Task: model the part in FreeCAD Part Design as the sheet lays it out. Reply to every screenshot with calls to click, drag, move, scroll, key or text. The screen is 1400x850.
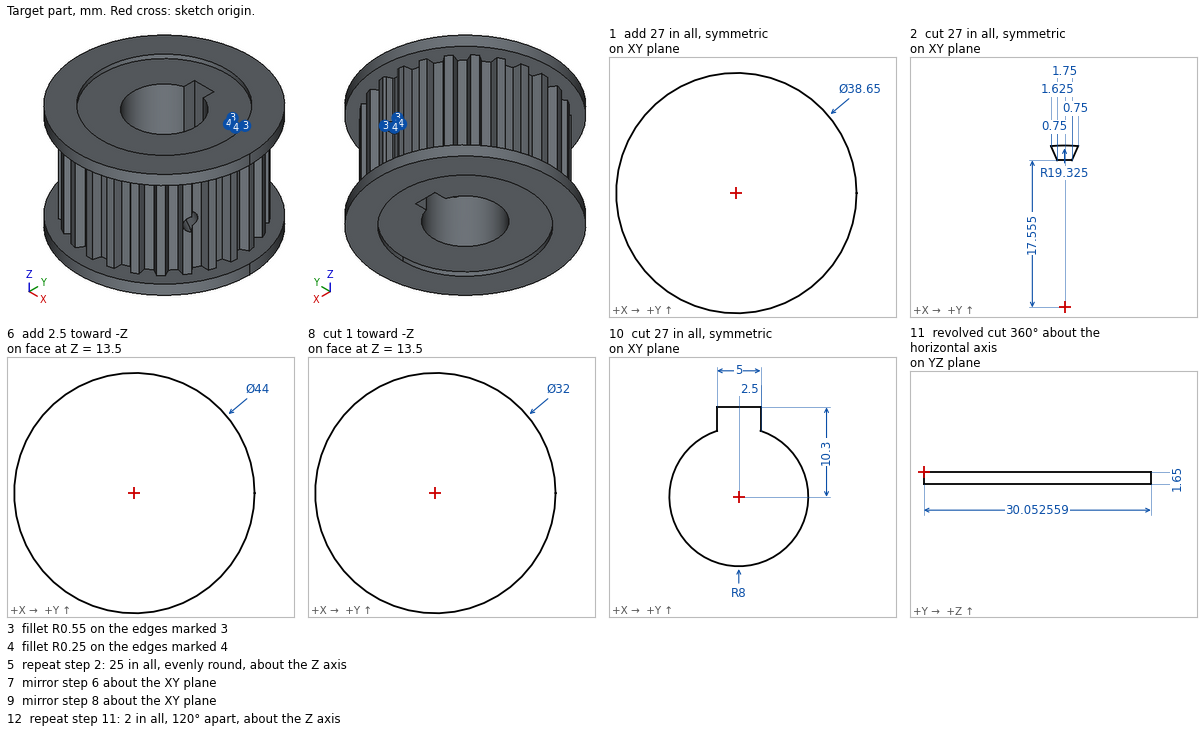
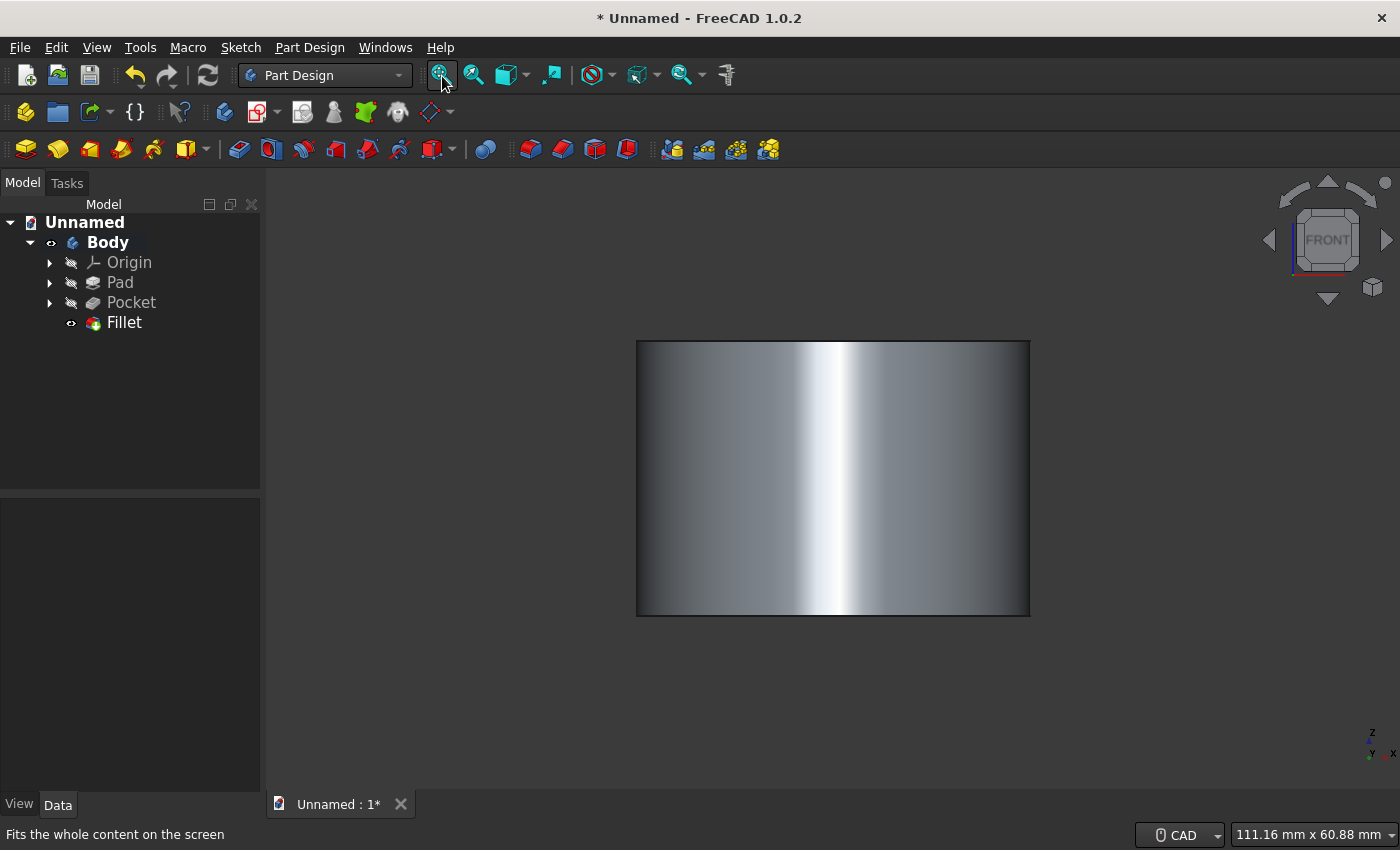
click(442, 76)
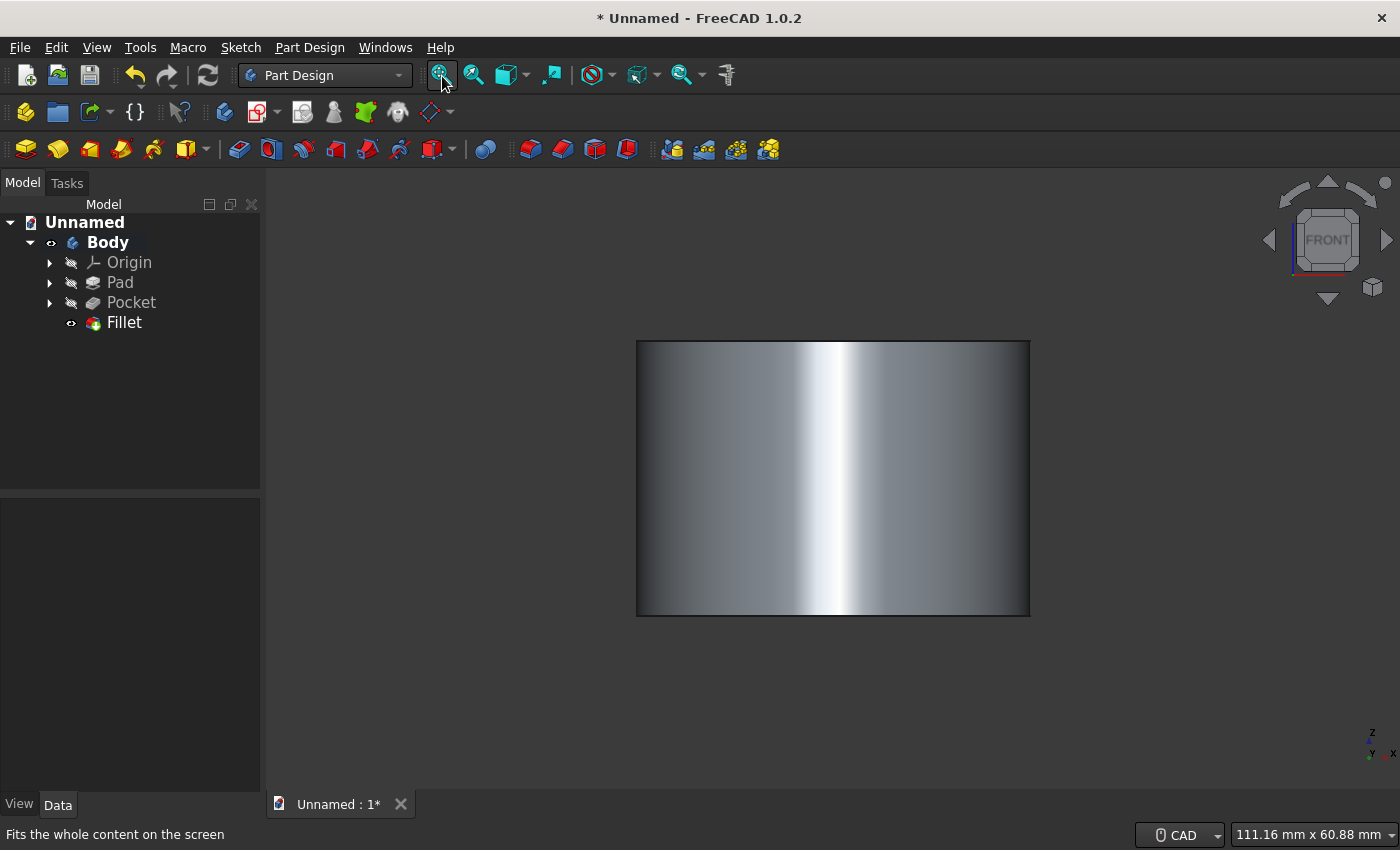
key(3)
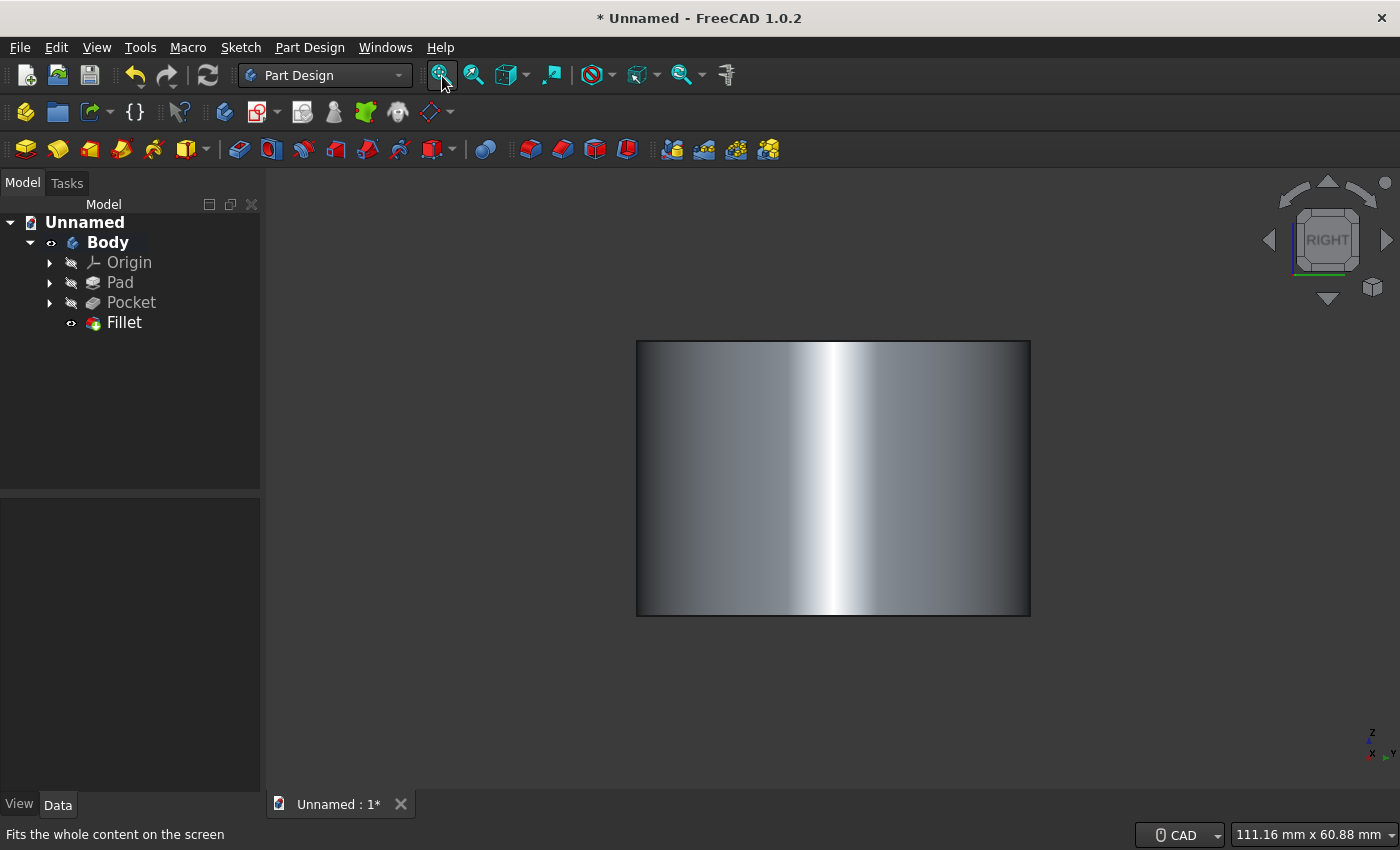
click(442, 76)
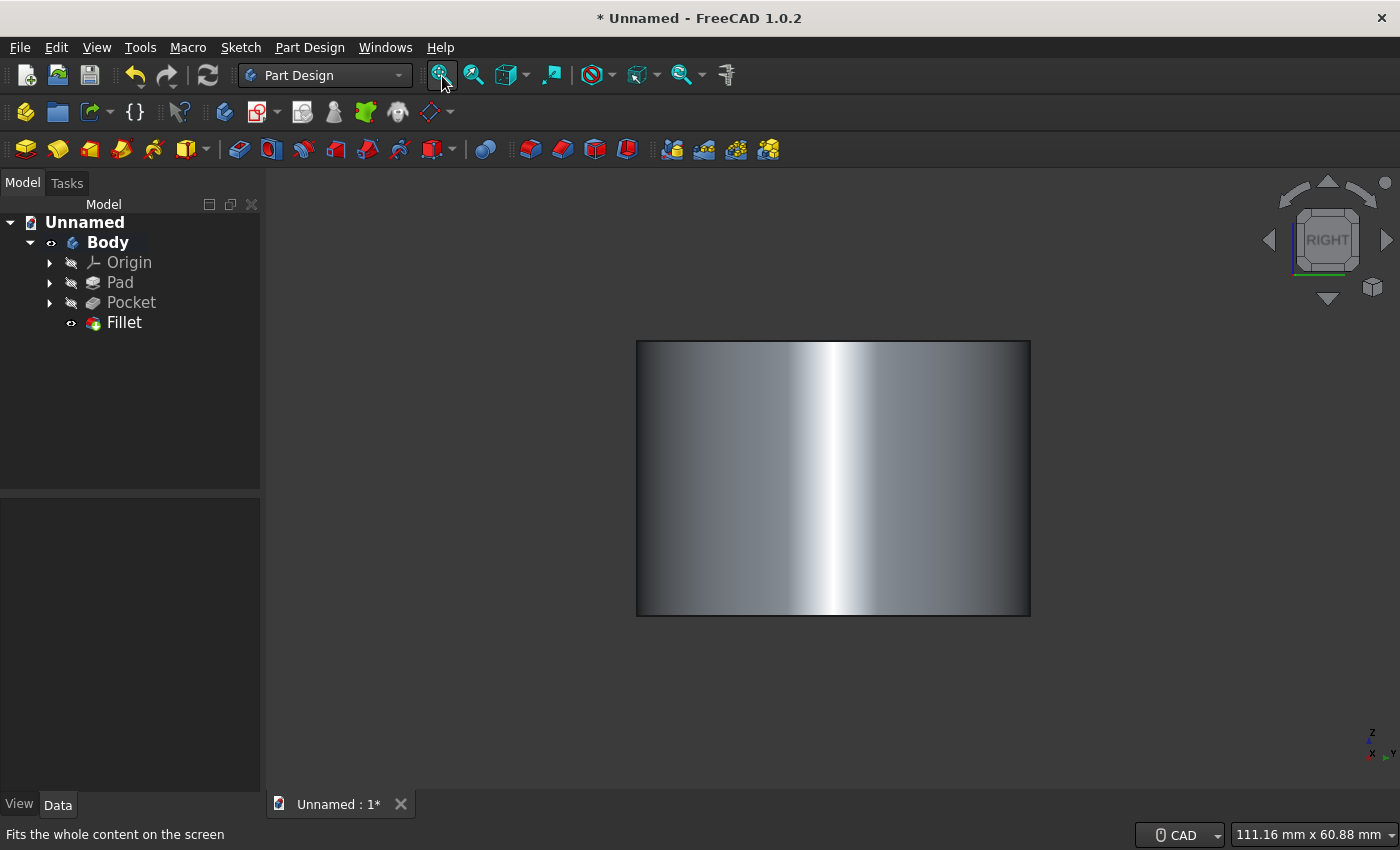
key(5)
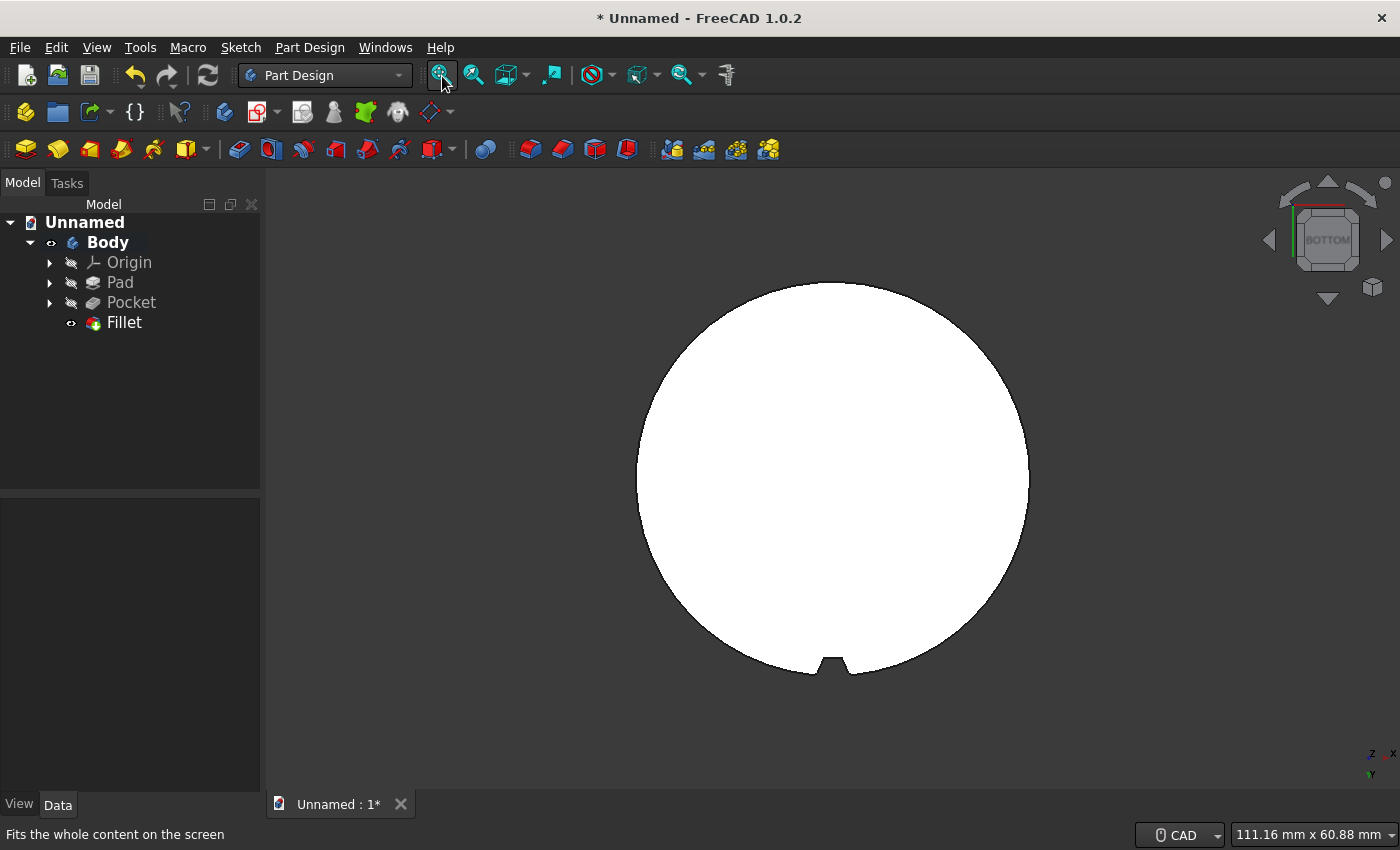
key(4)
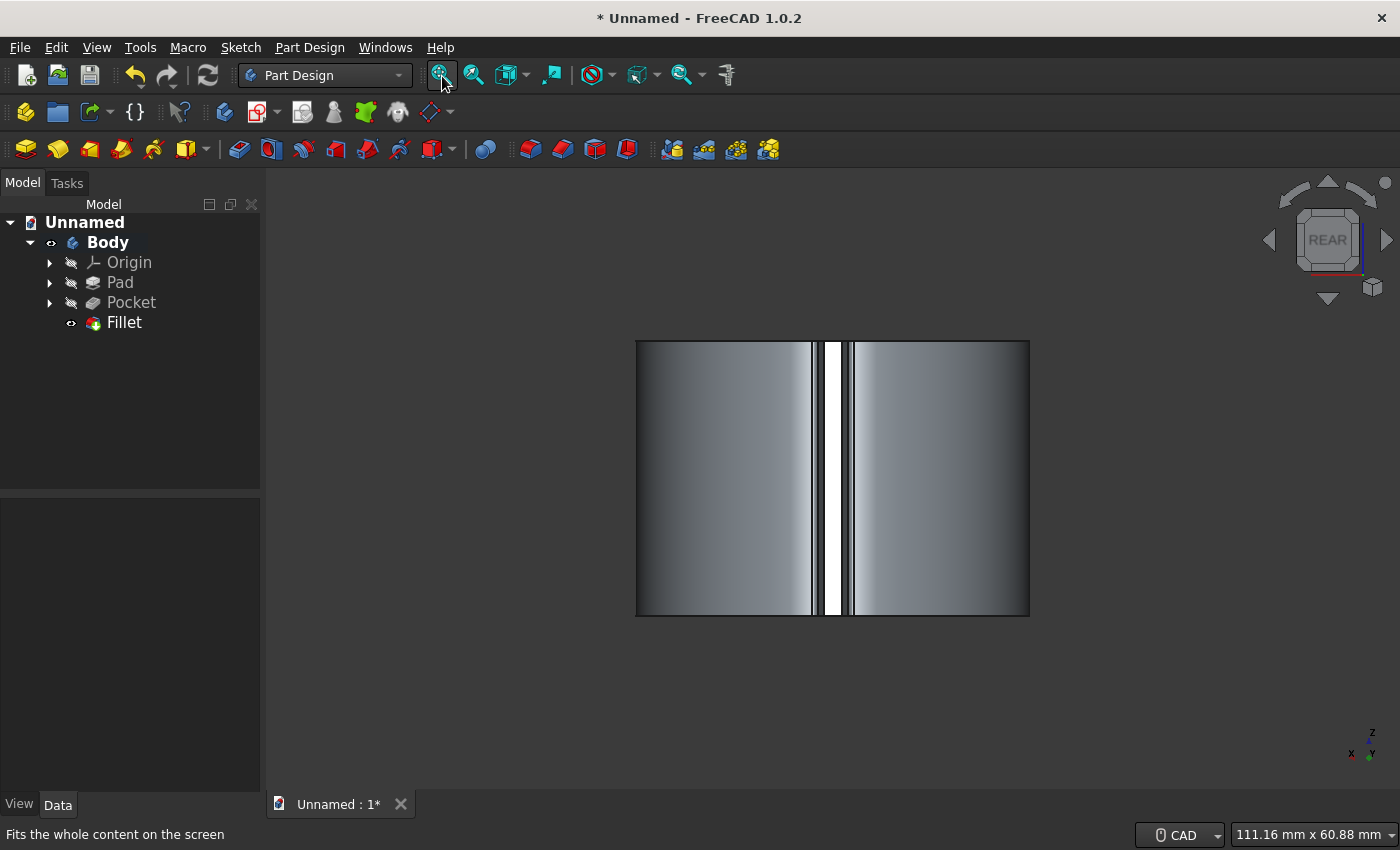
click(442, 76)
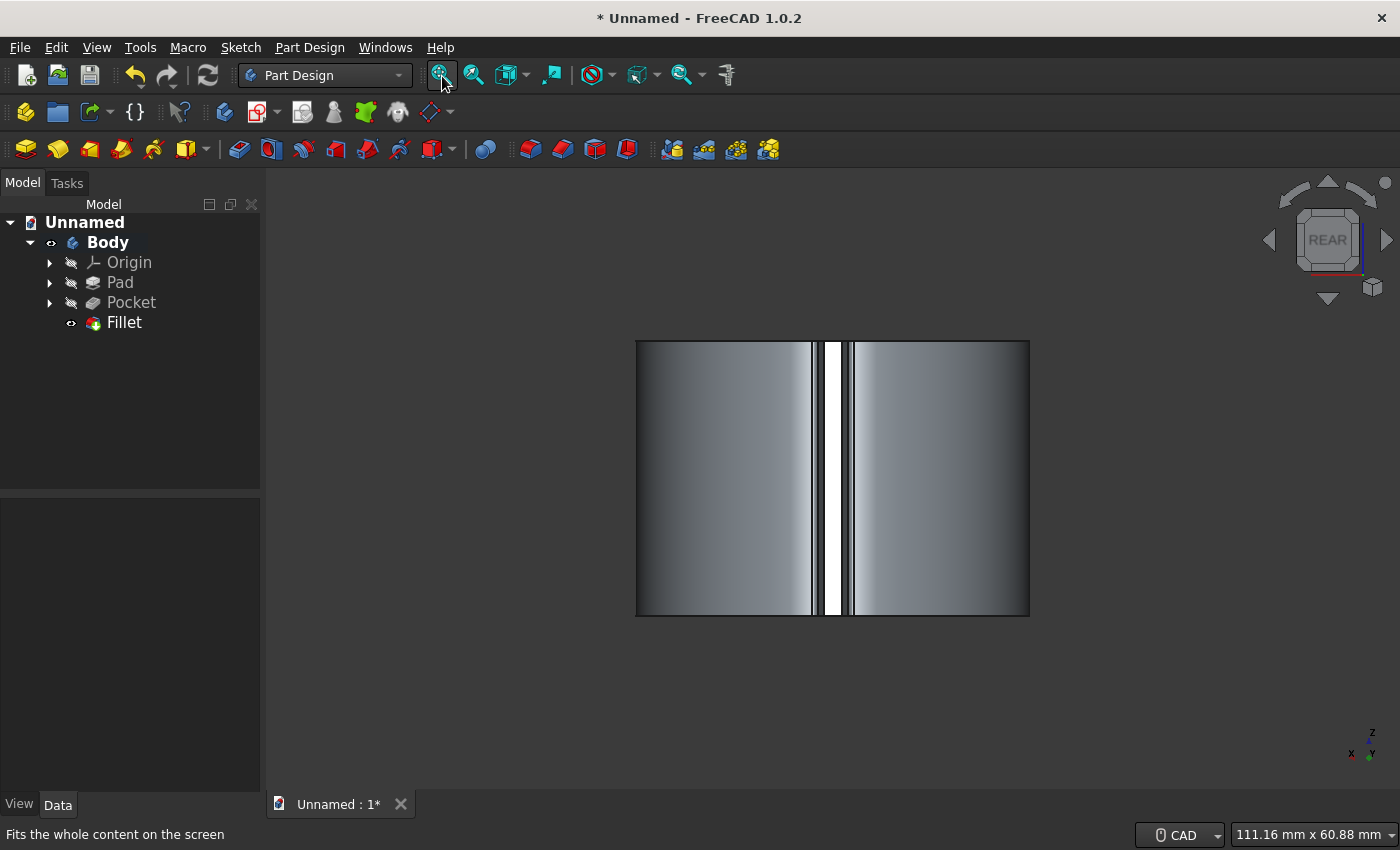
key(6)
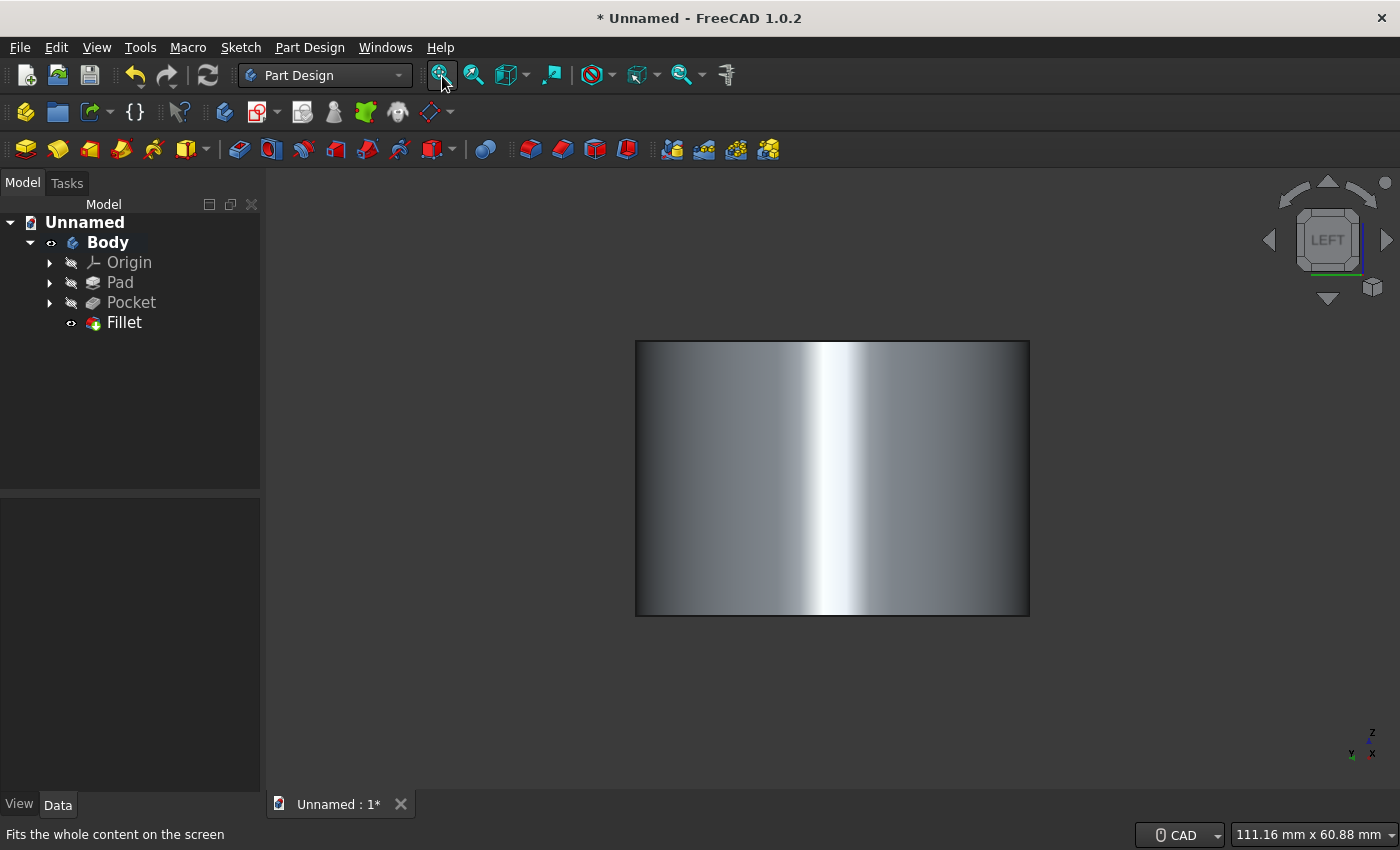
click(442, 76)